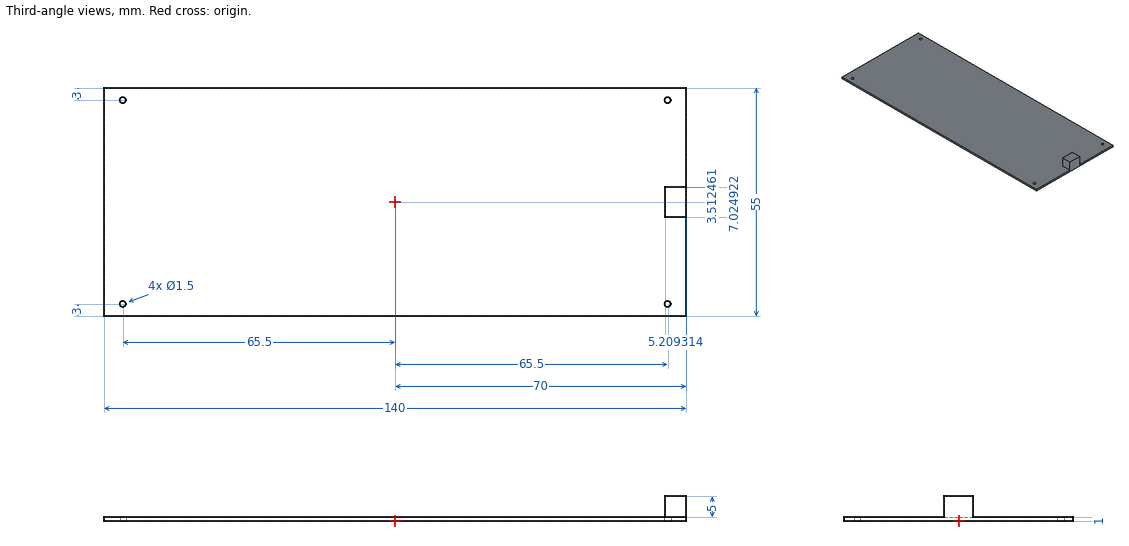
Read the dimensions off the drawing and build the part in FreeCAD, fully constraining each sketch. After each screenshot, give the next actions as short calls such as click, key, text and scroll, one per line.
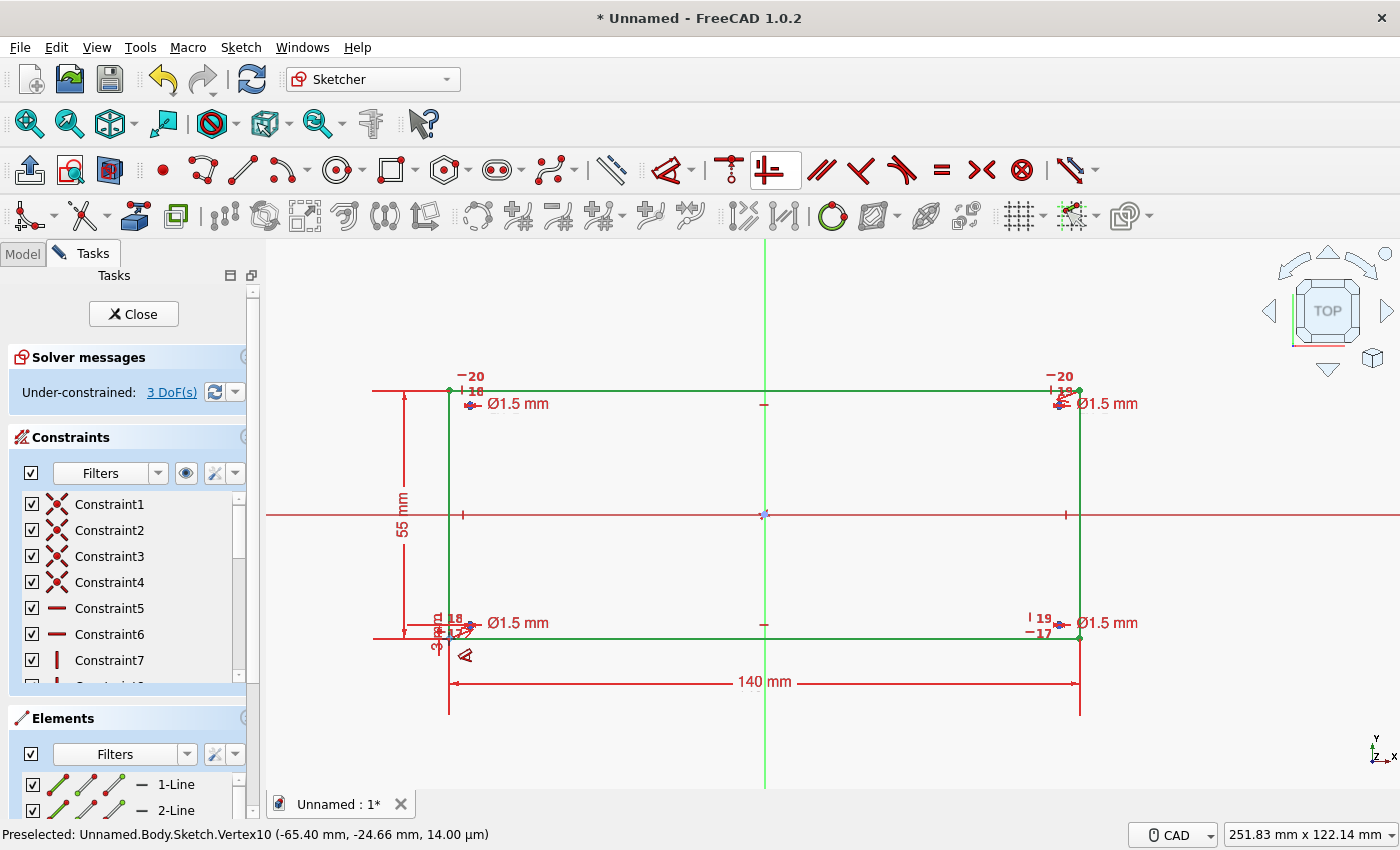
scroll(449, 391, up, 6)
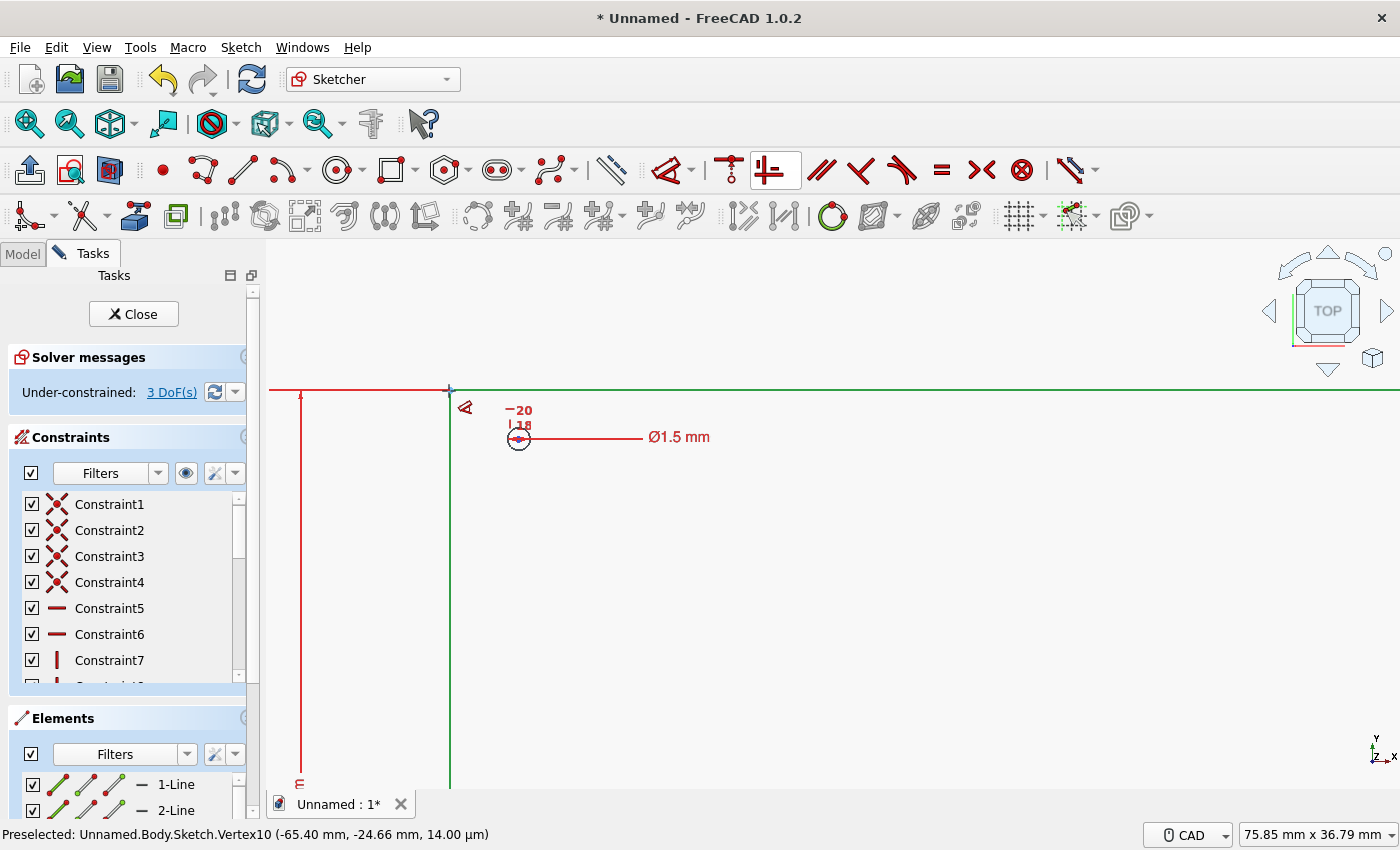
click(450, 390)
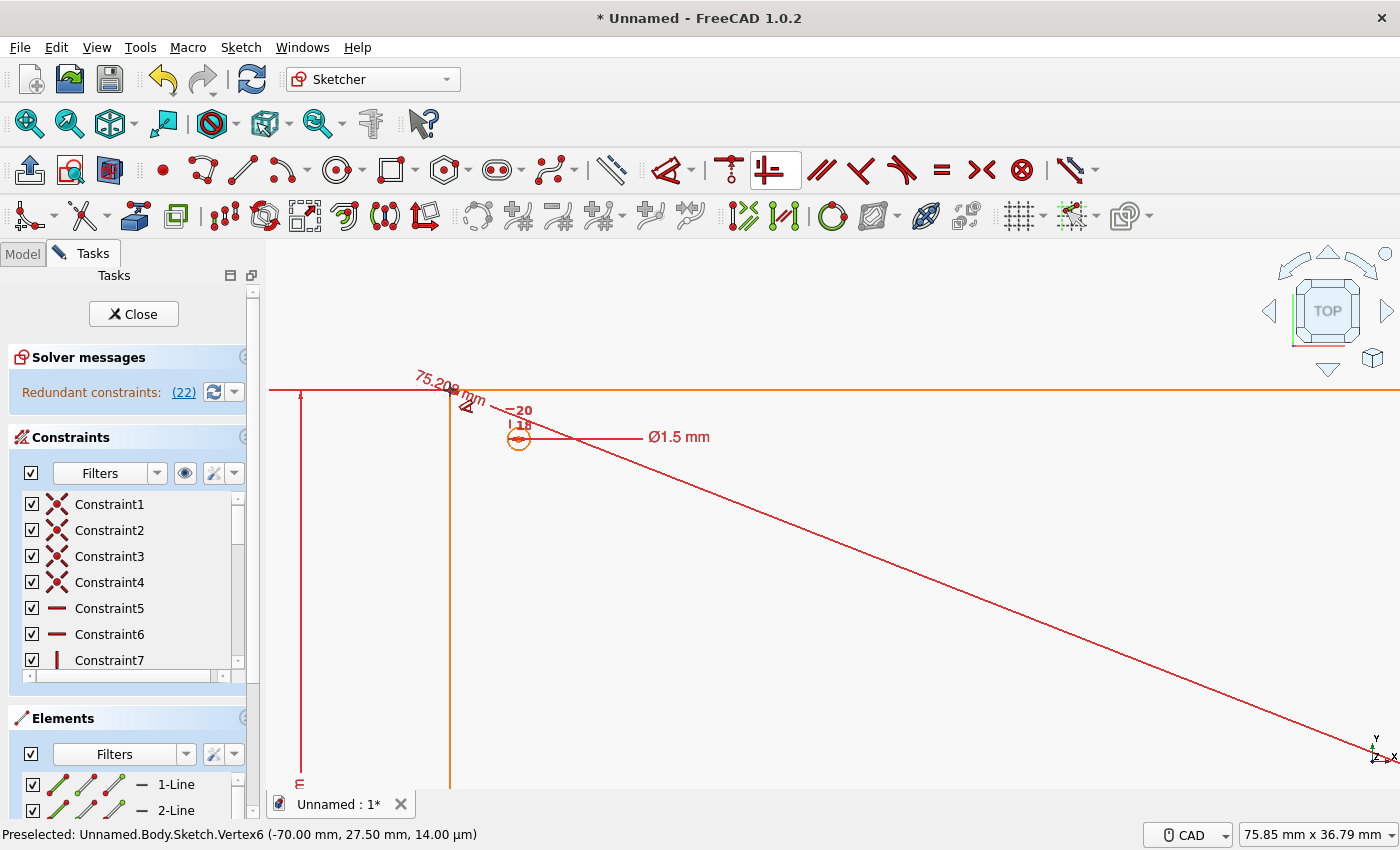
click(519, 439)
click(416, 415)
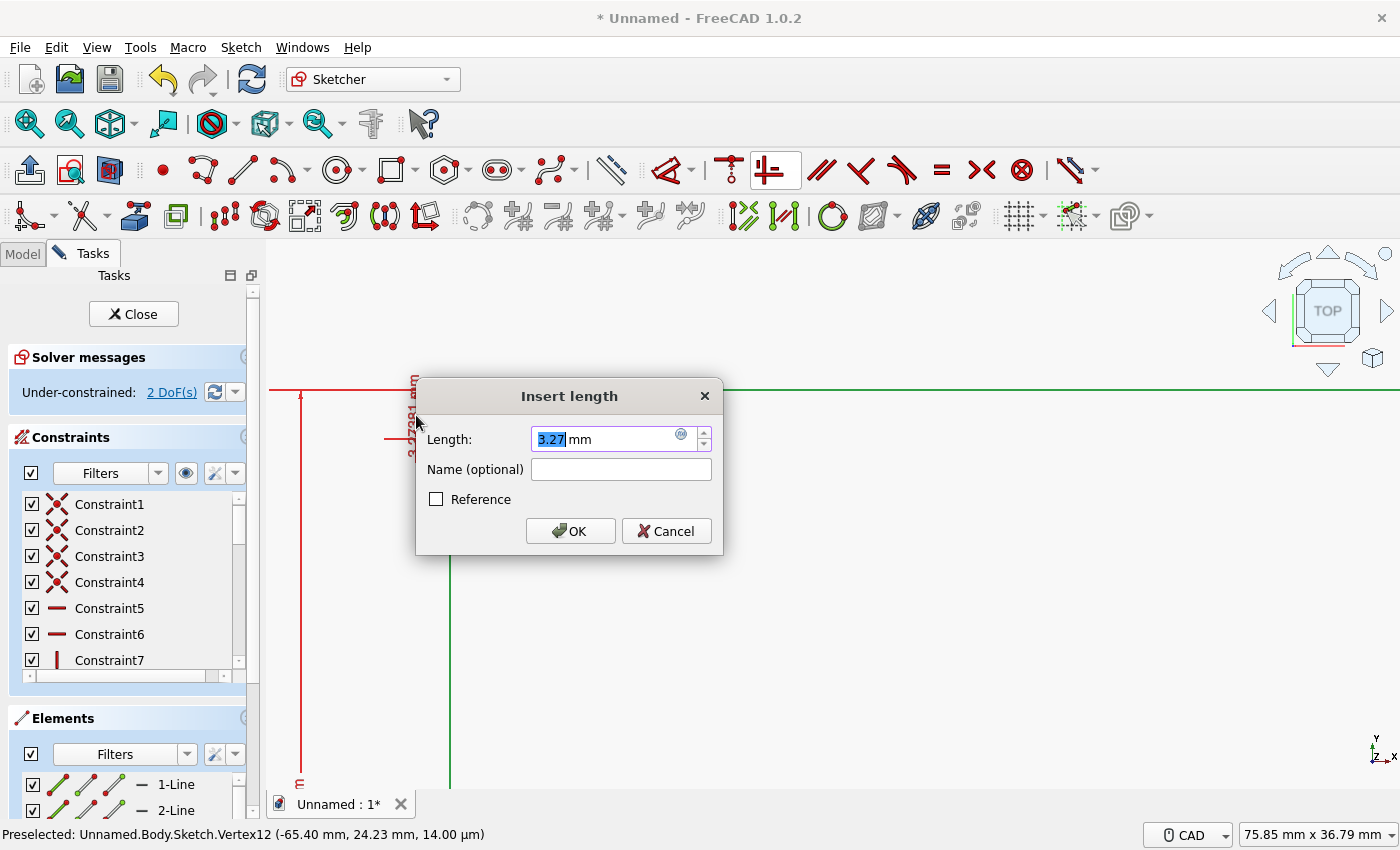
text(3)
key(Return)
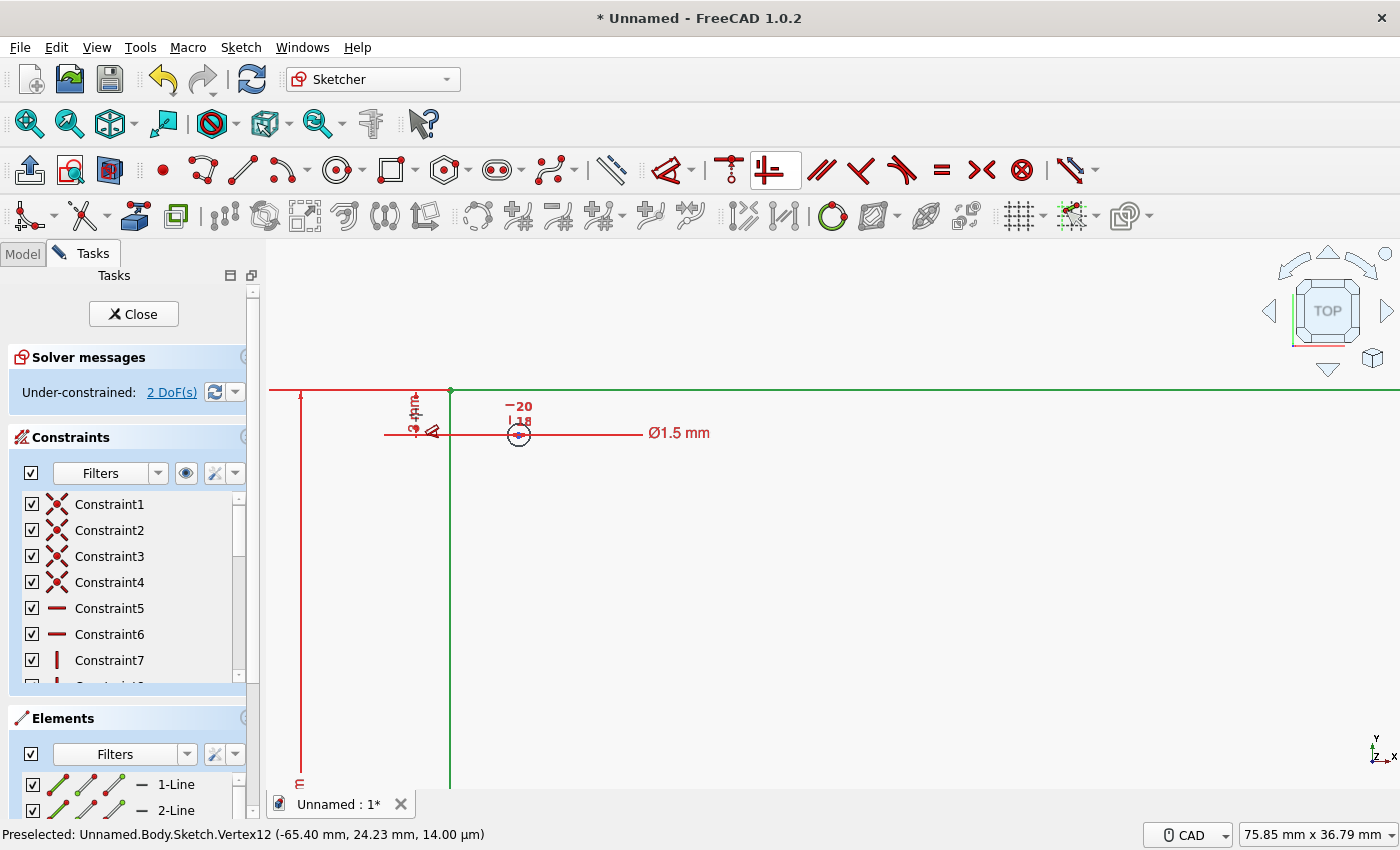
scroll(449, 390, down, 6)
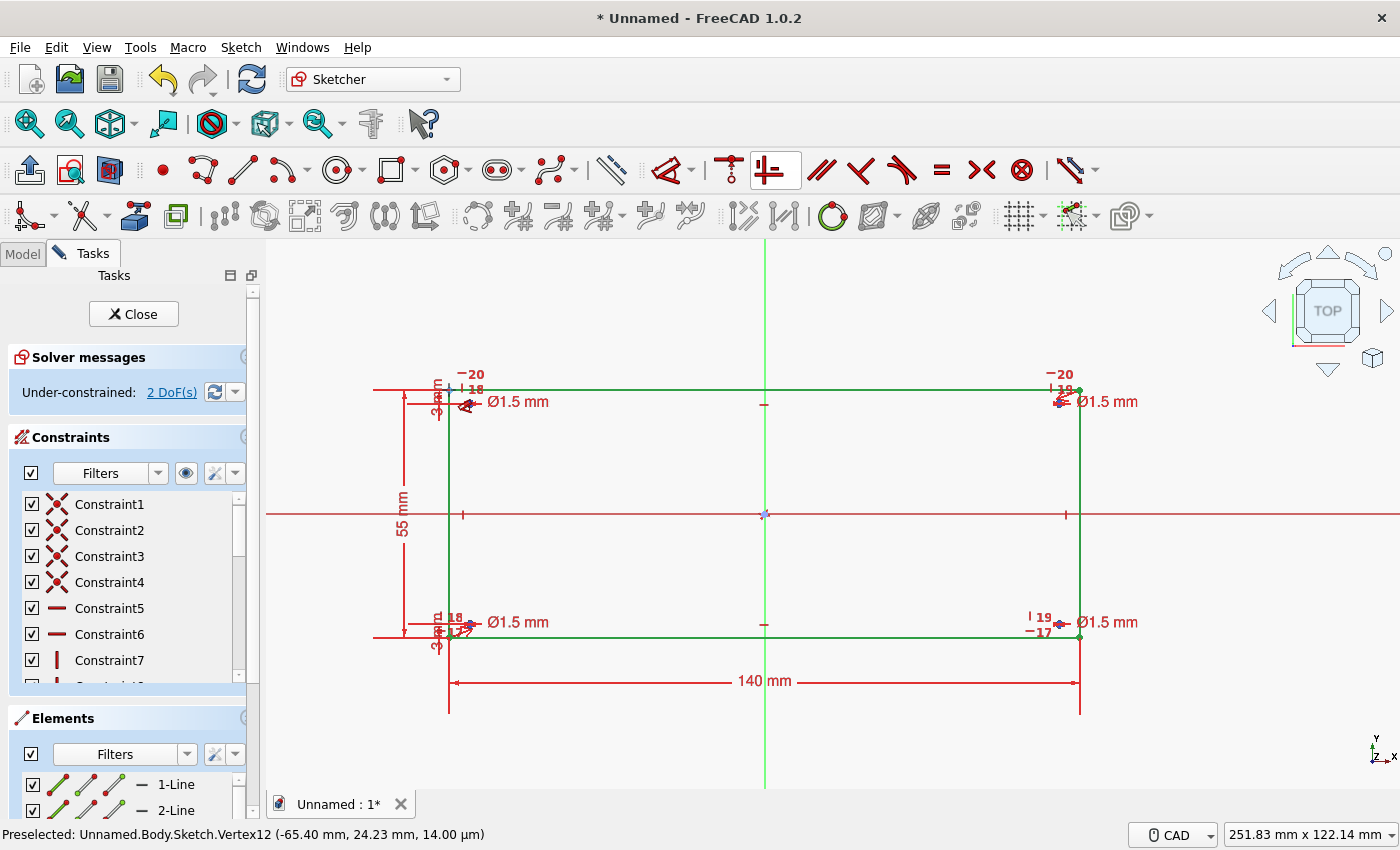
click(470, 624)
click(617, 658)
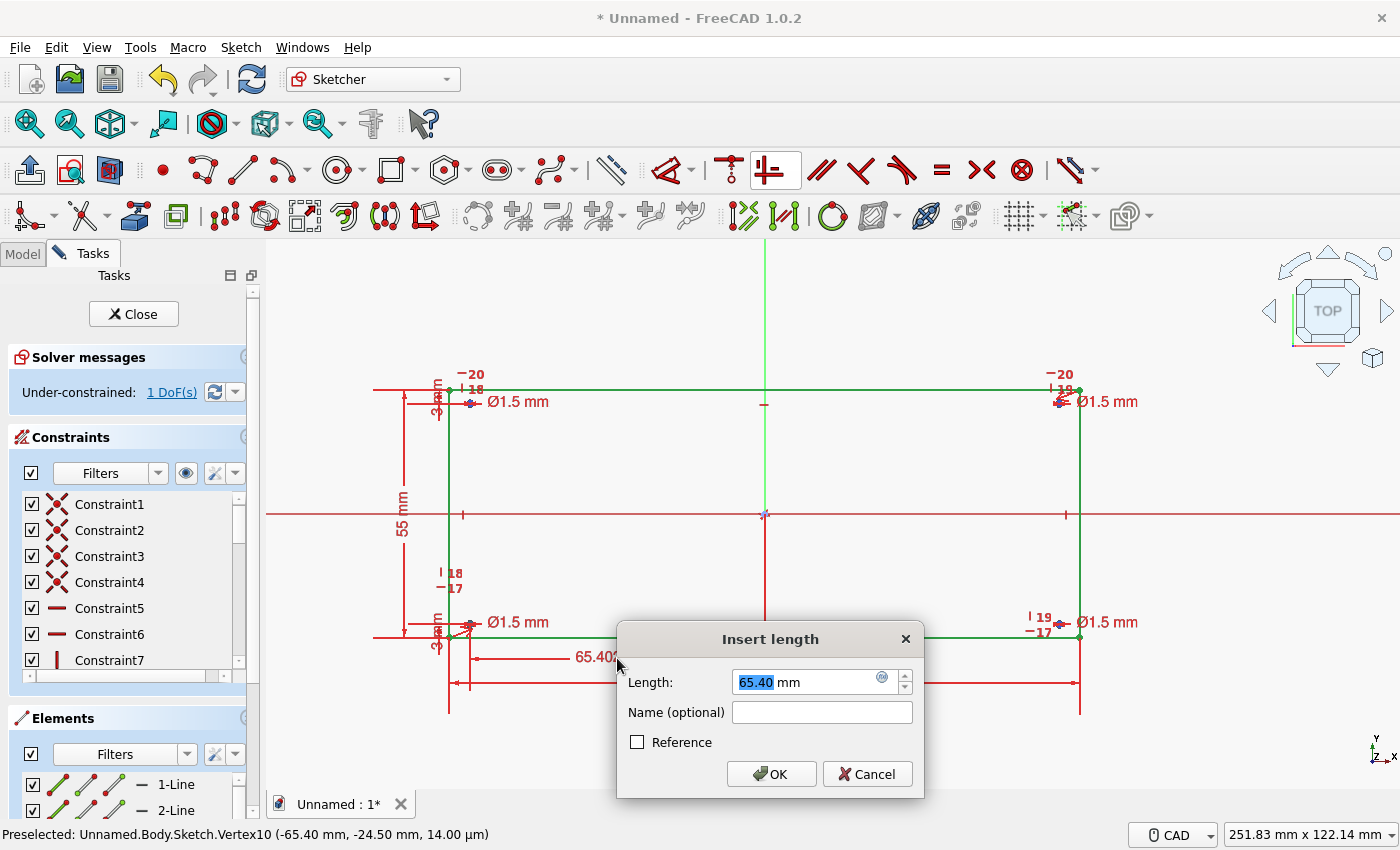
text(65.5)
key(Return)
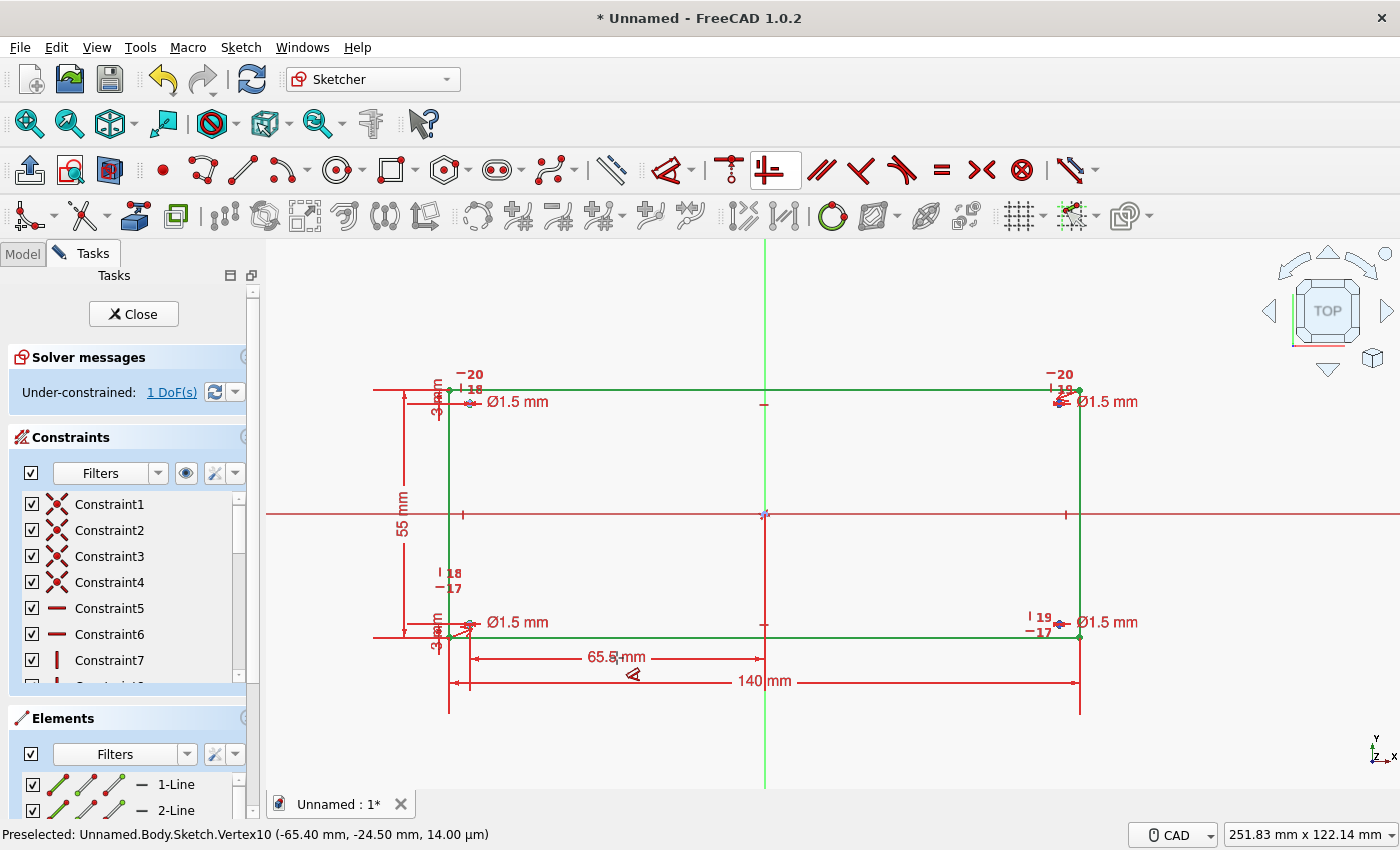
click(1059, 624)
click(912, 658)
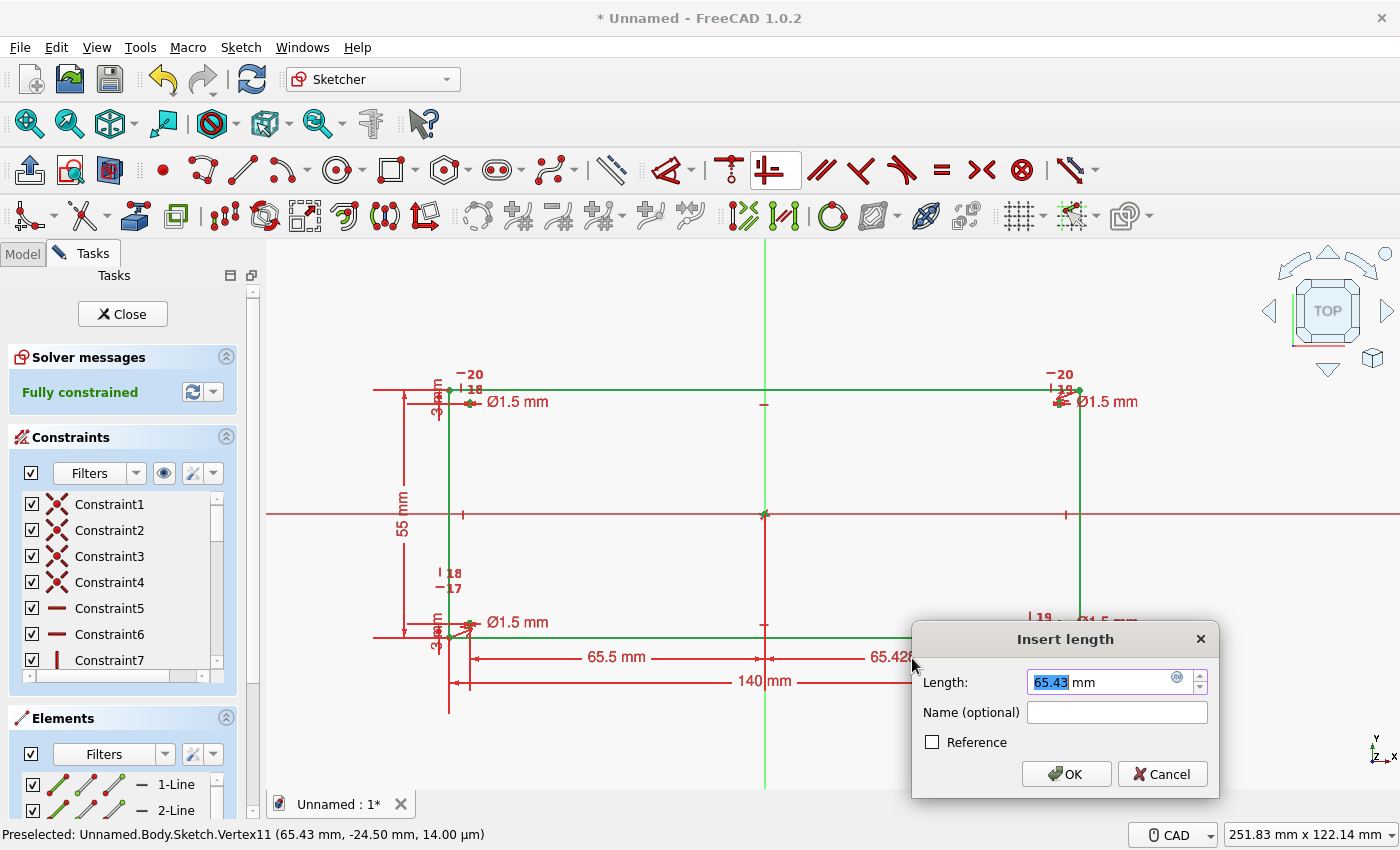
text(65.5)
key(Return)
key(Escape)